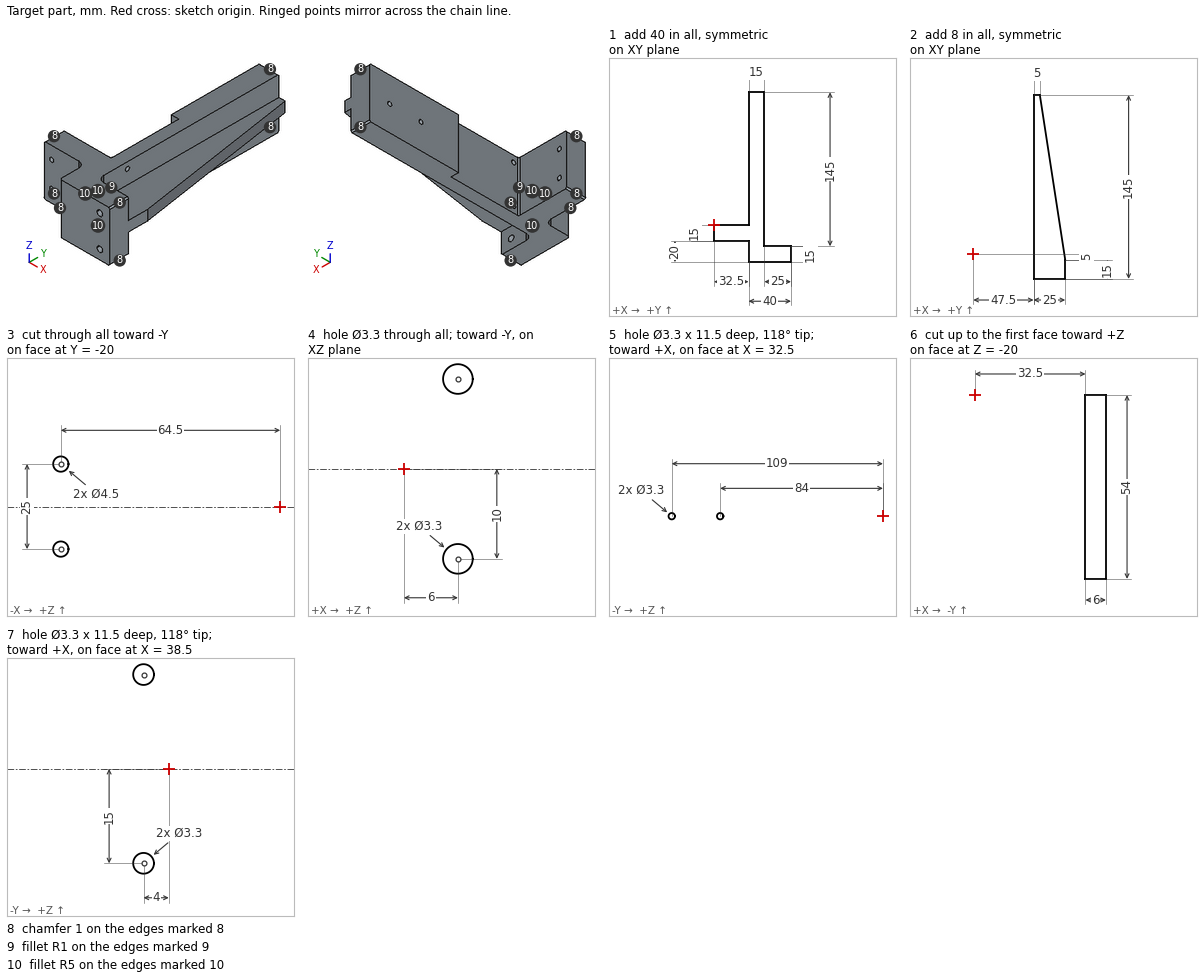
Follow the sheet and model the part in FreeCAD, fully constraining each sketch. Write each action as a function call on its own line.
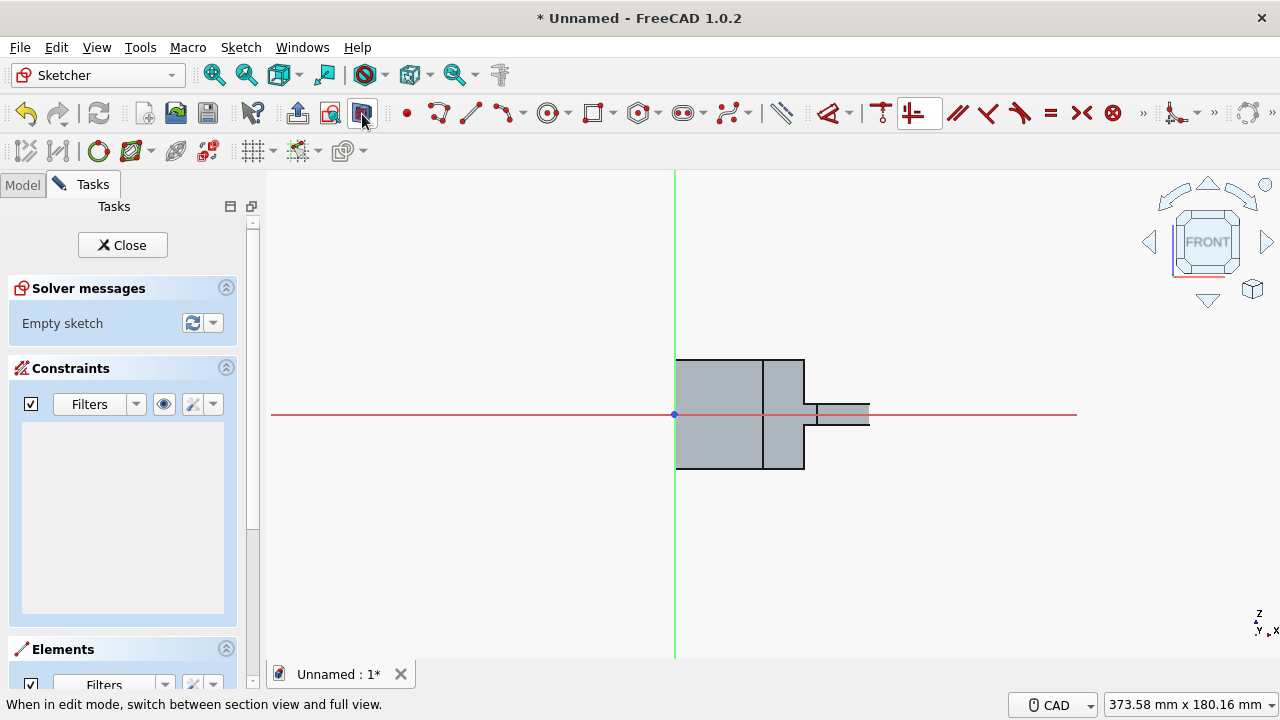
scroll(680, 414, up, 8)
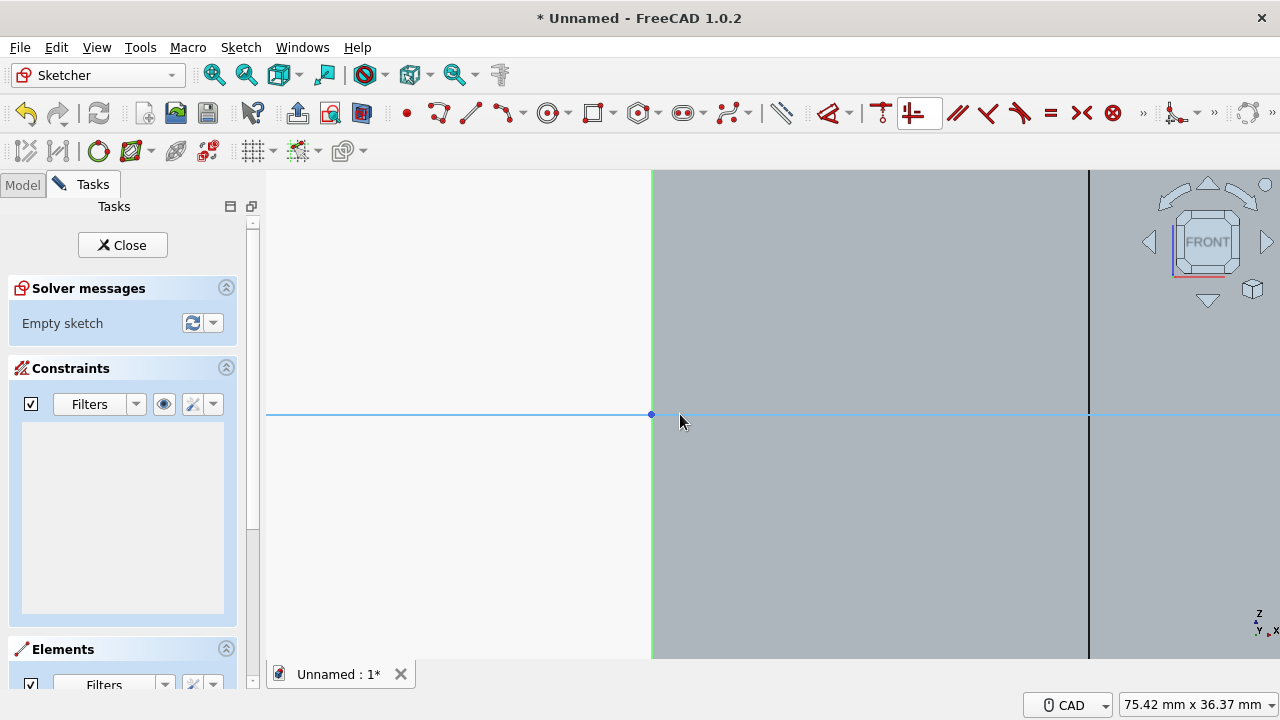
click(548, 114)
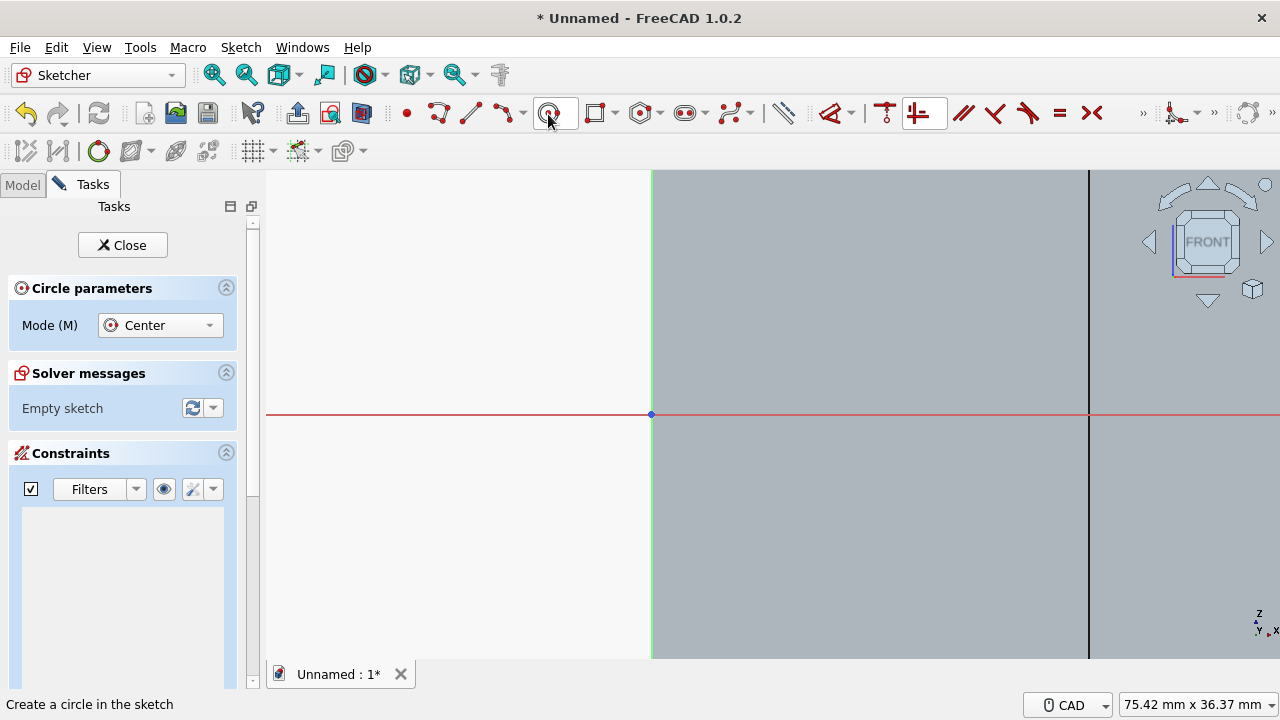
click(732, 549)
click(748, 533)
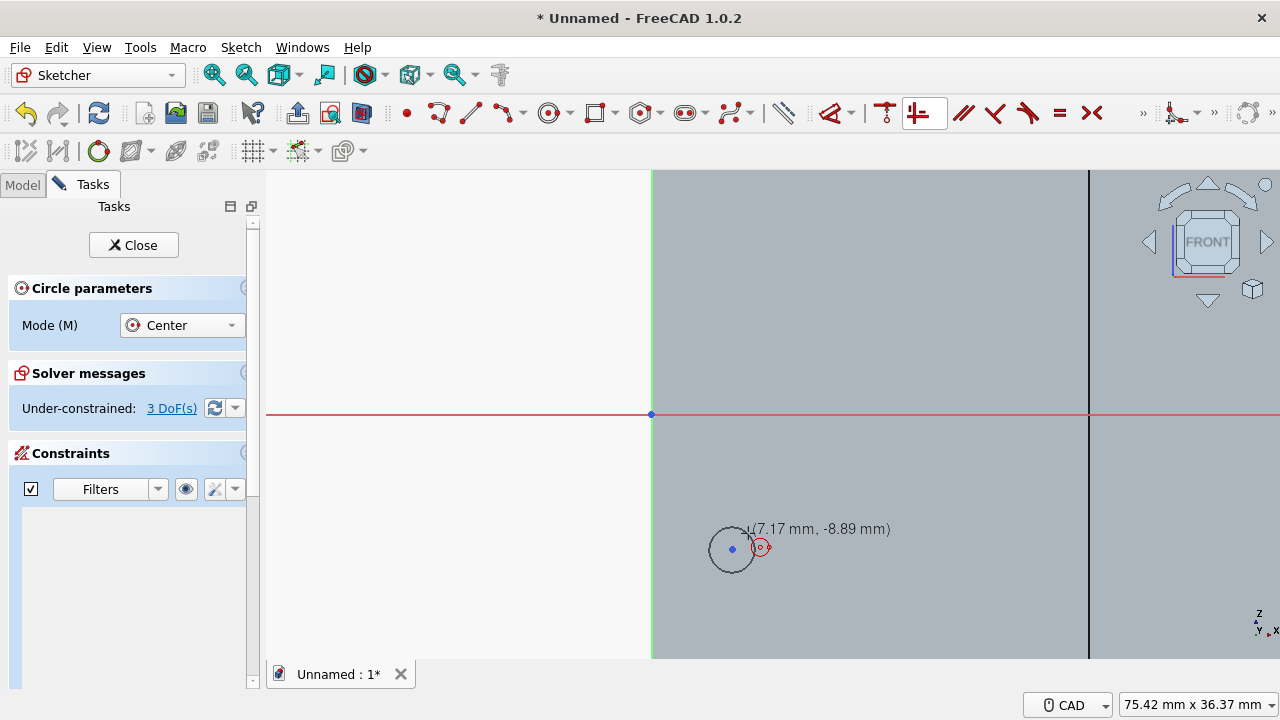
click(732, 280)
click(748, 264)
key(Escape)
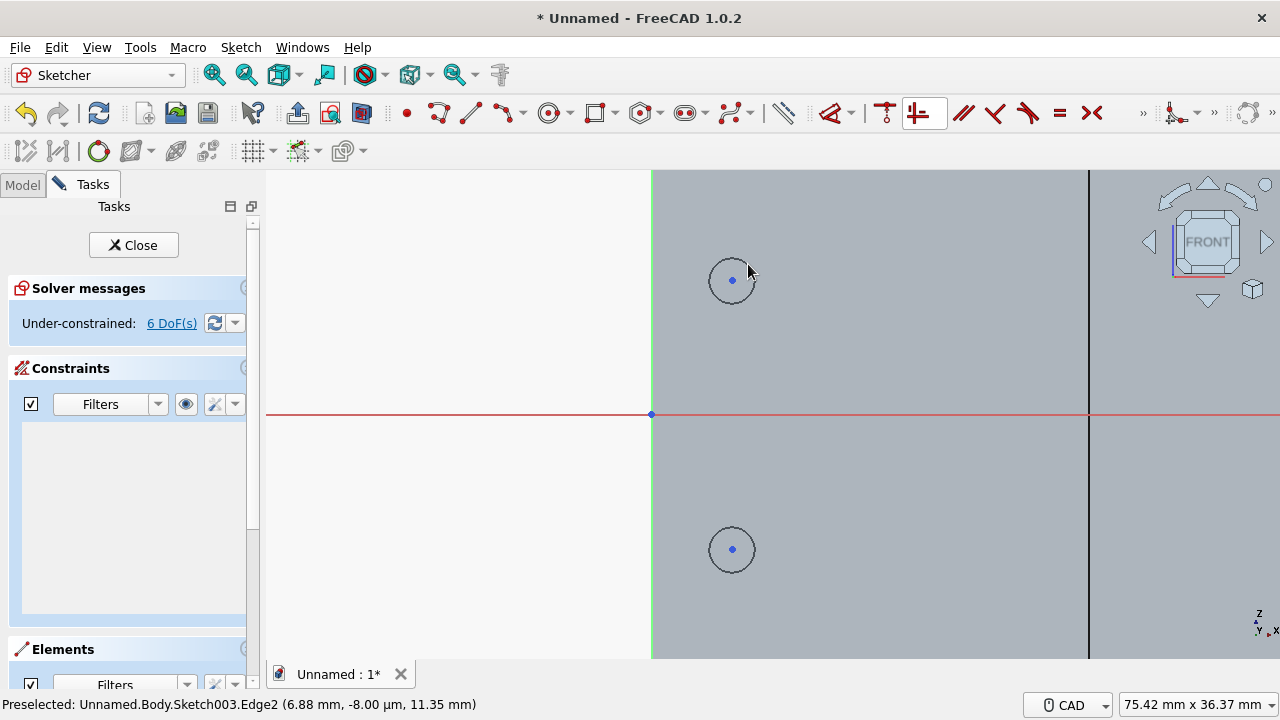
click(748, 534)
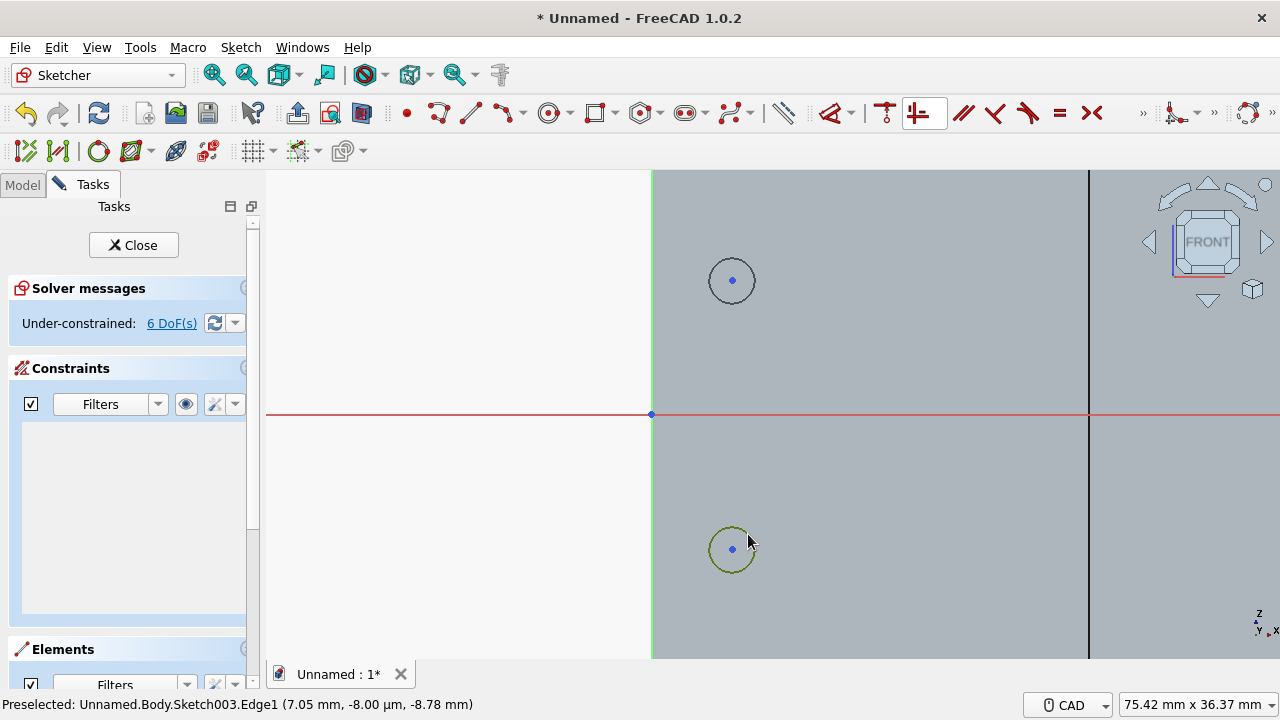
click(748, 265)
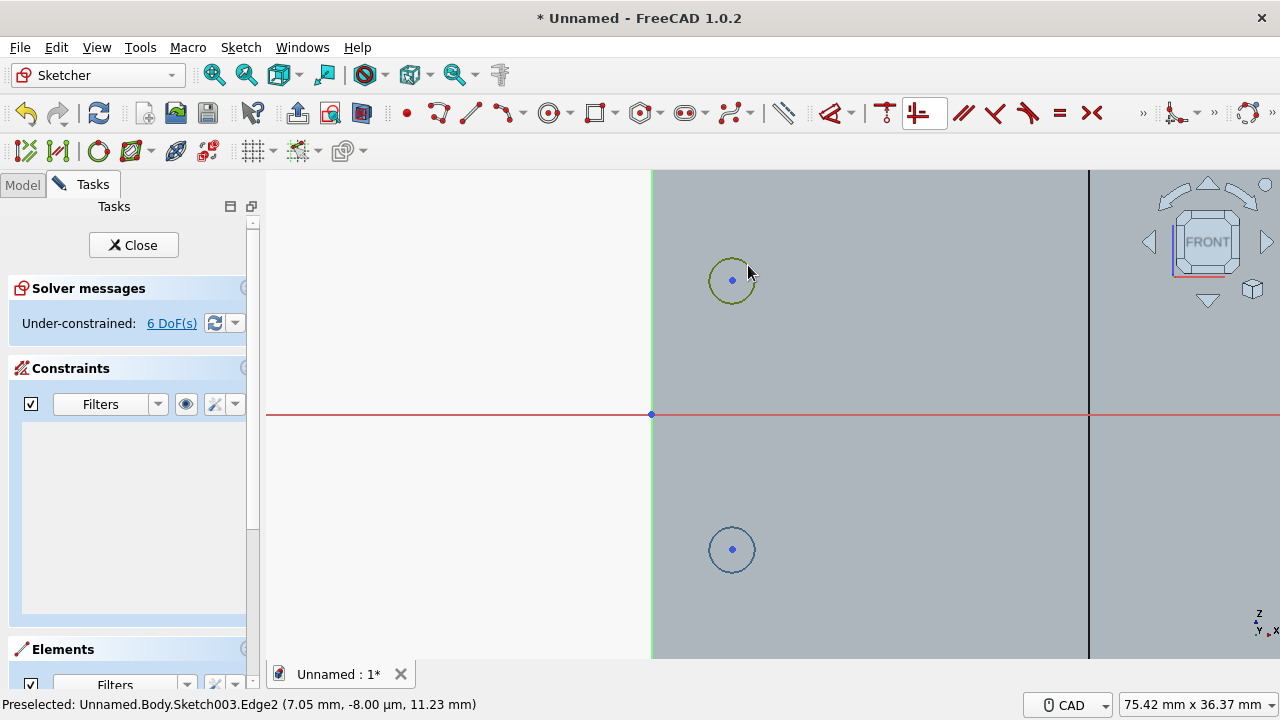
click(1060, 114)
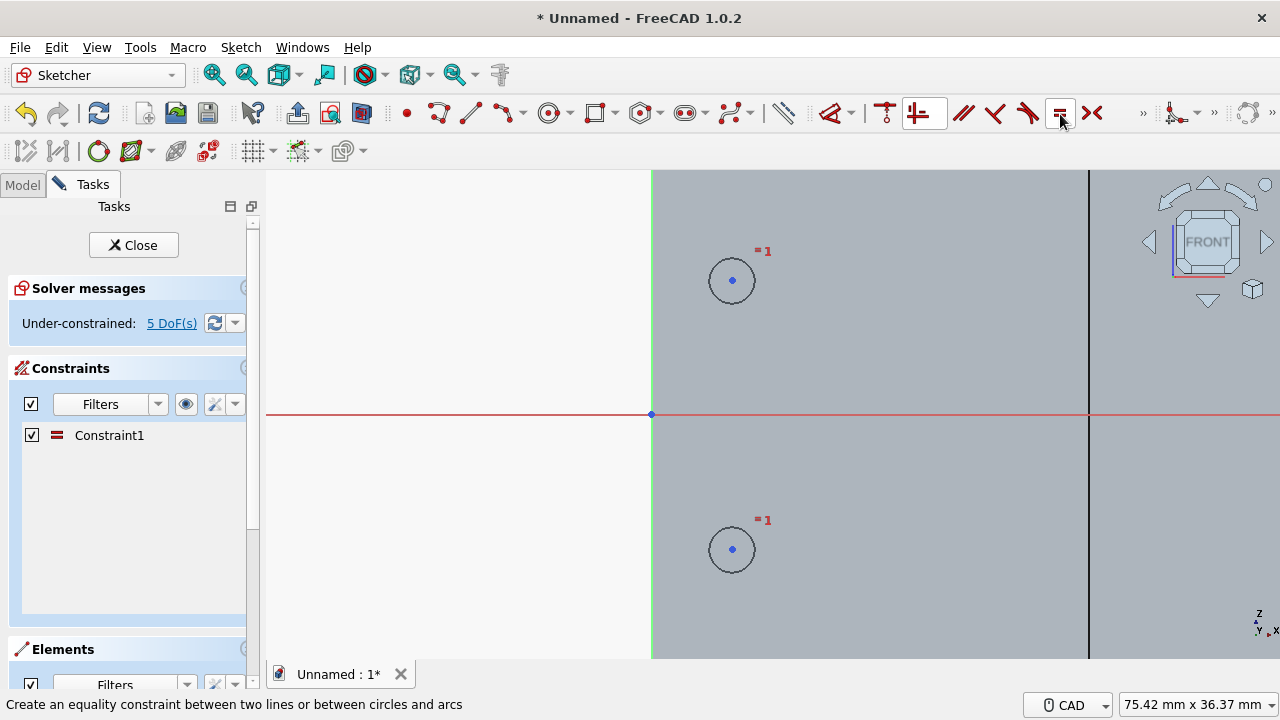
click(732, 550)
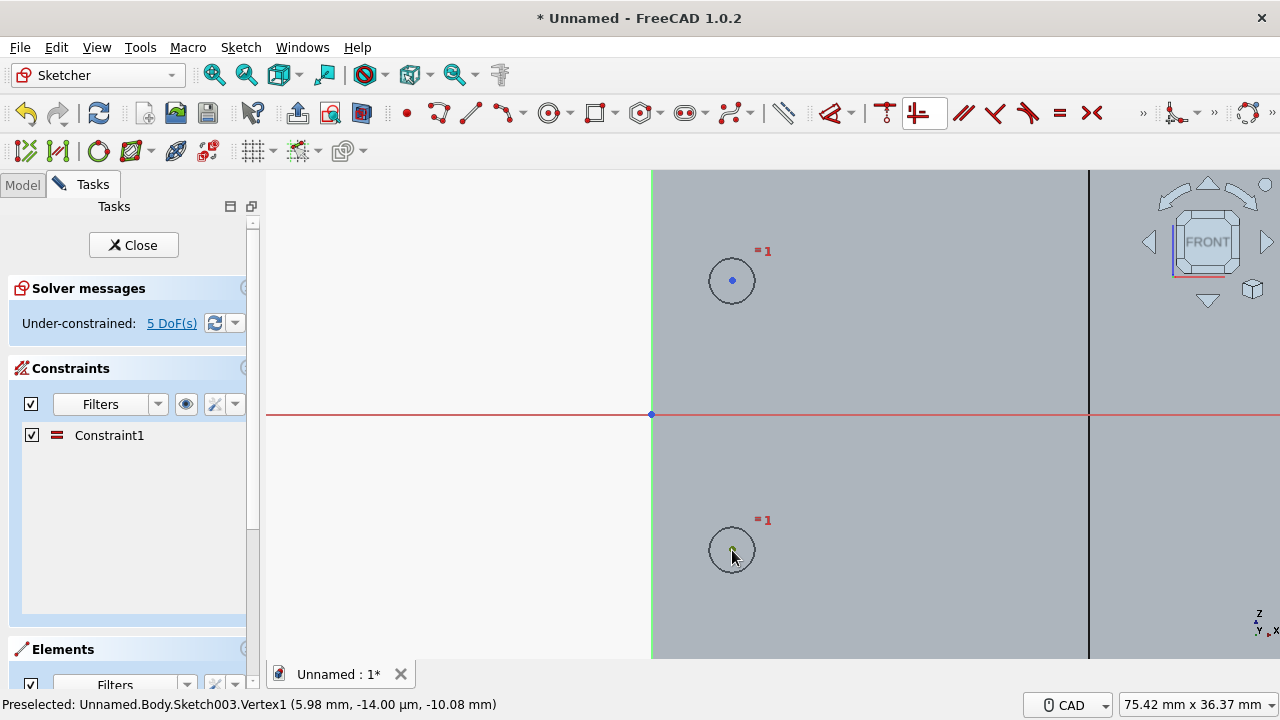
click(732, 281)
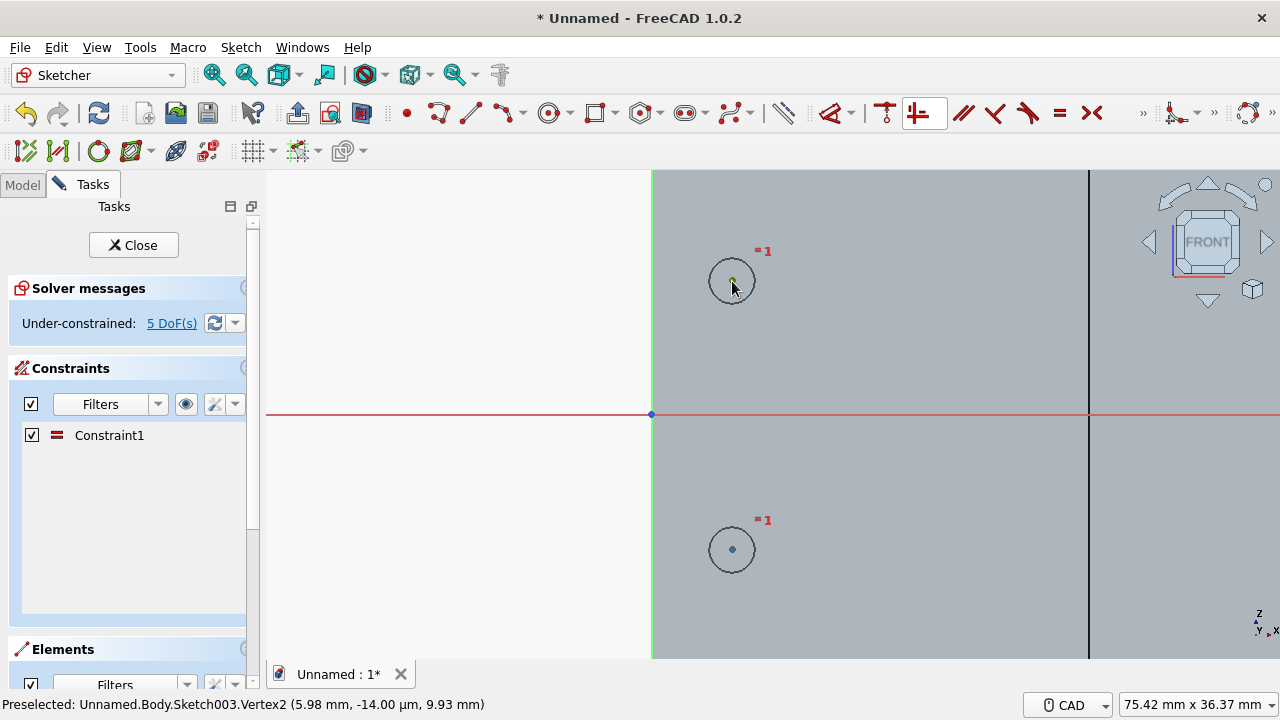
click(353, 414)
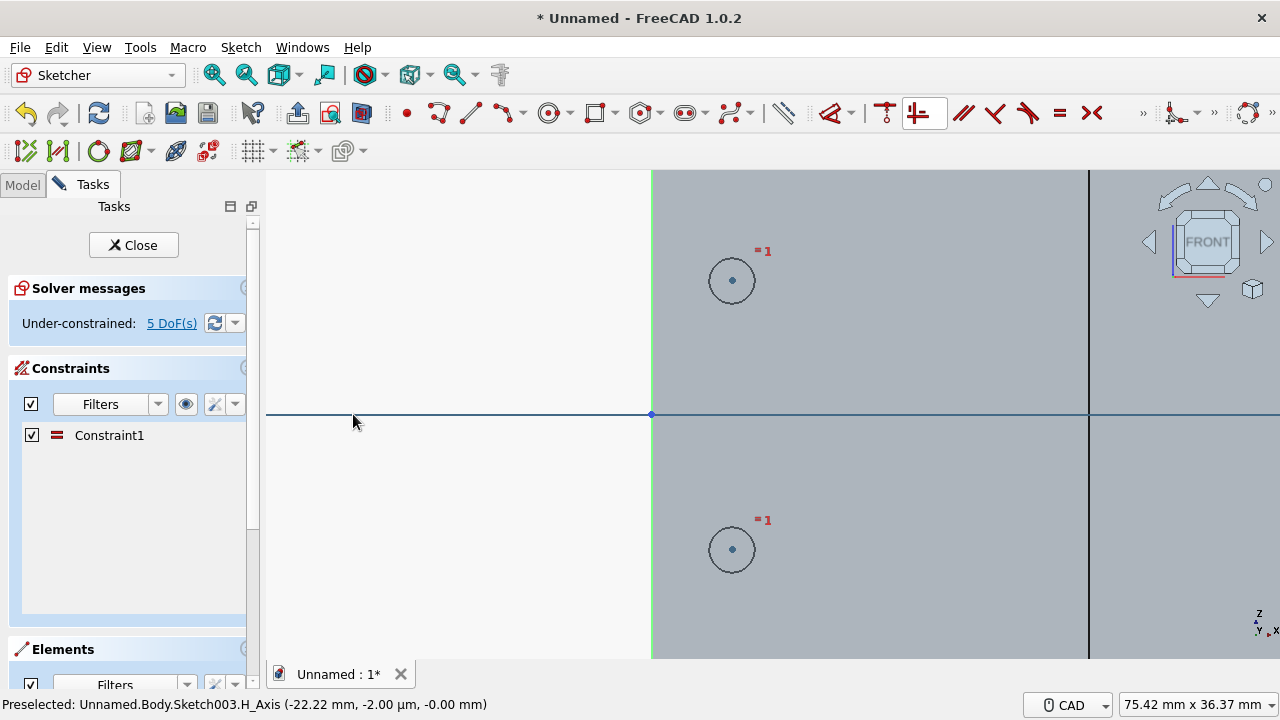
click(1092, 114)